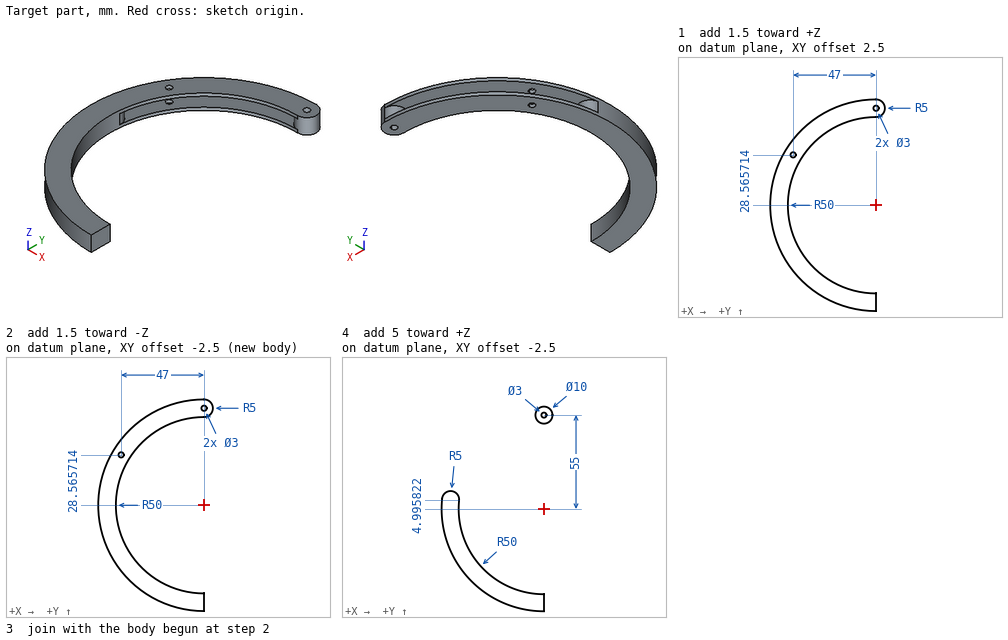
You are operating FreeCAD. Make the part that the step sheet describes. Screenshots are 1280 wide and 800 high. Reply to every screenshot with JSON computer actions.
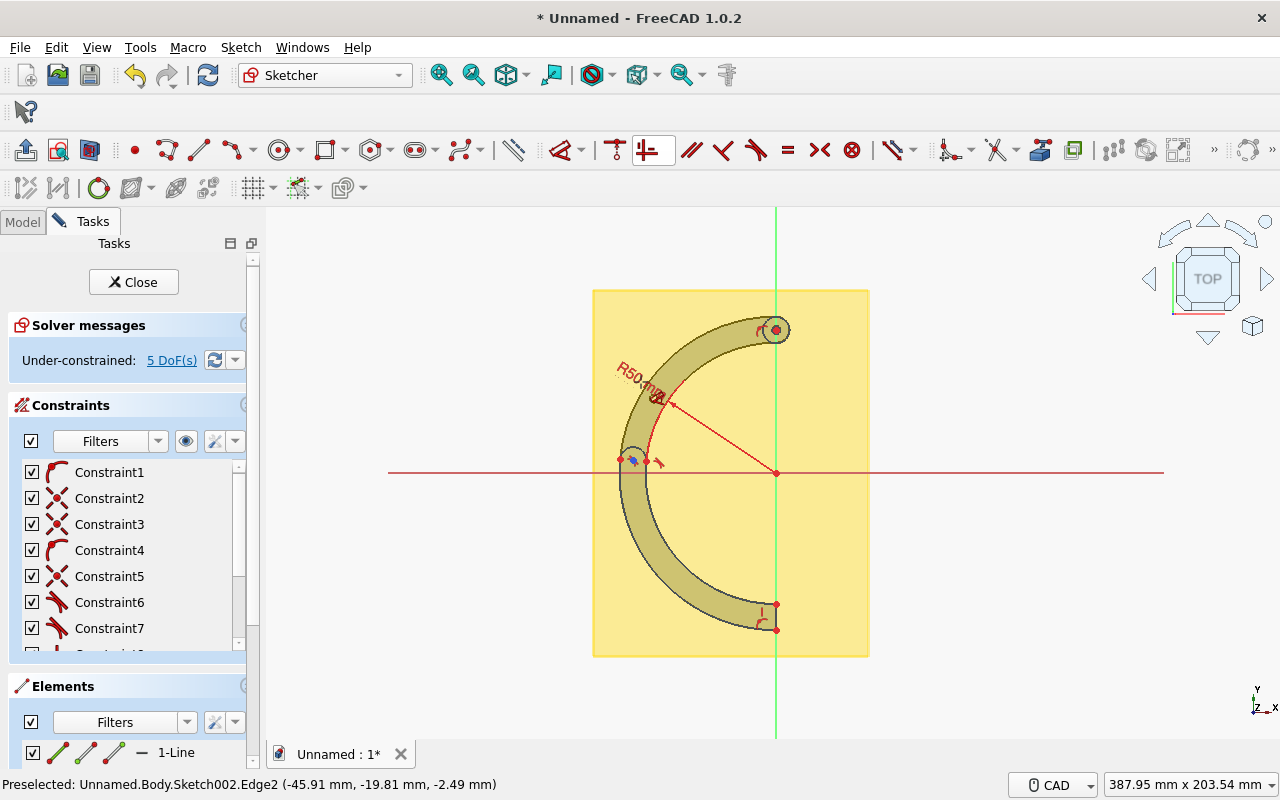
{"action": "scroll", "coordinate": [642, 450], "scroll_direction": "up", "scroll_amount": 6}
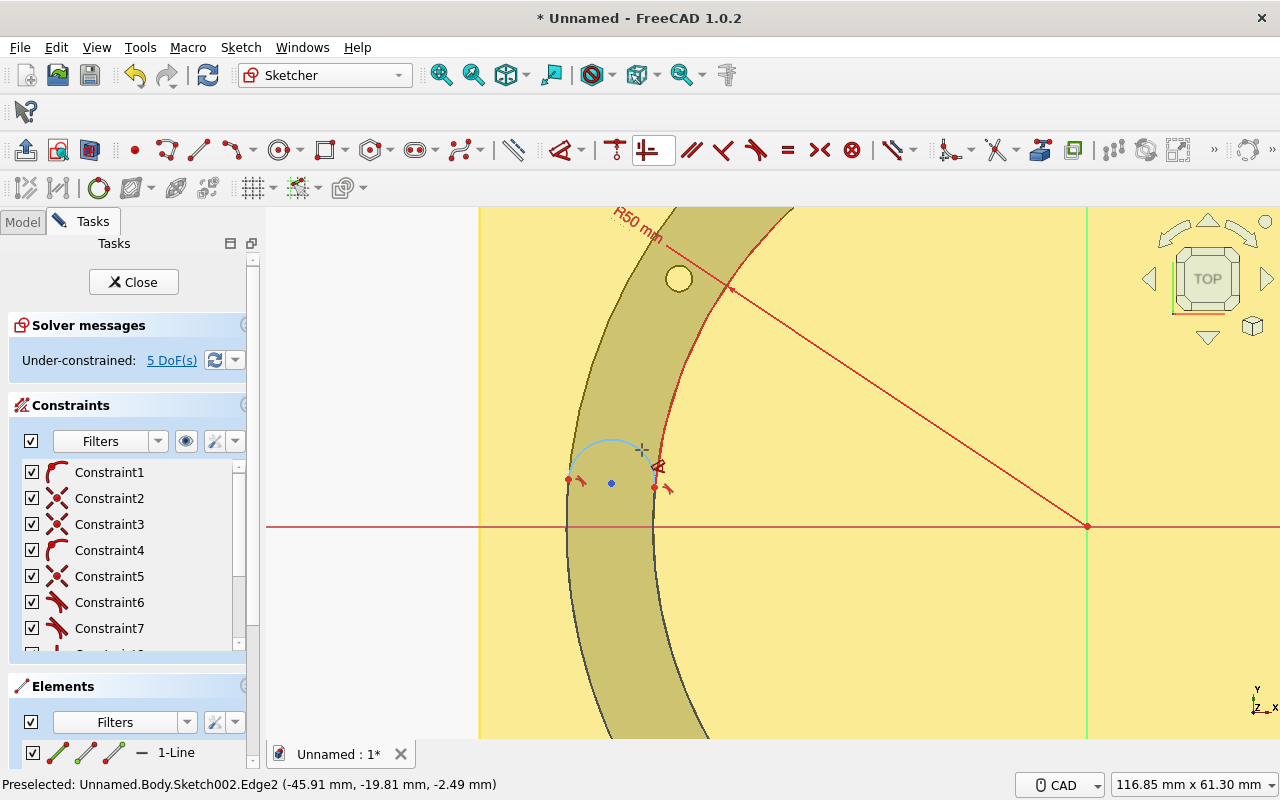
{"action": "left_click", "coordinate": [640, 450]}
{"action": "left_click", "coordinate": [661, 426]}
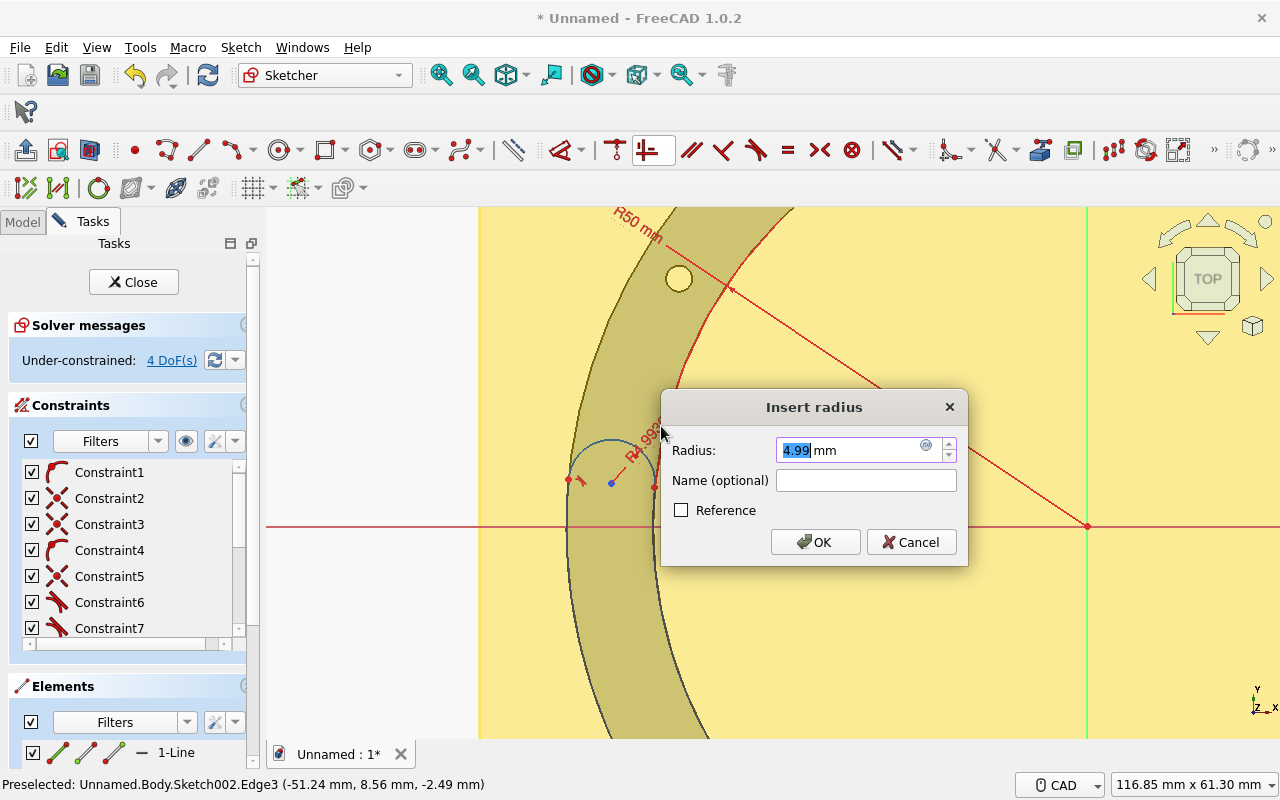
{"action": "type", "text": "5"}
{"action": "key", "text": "Return"}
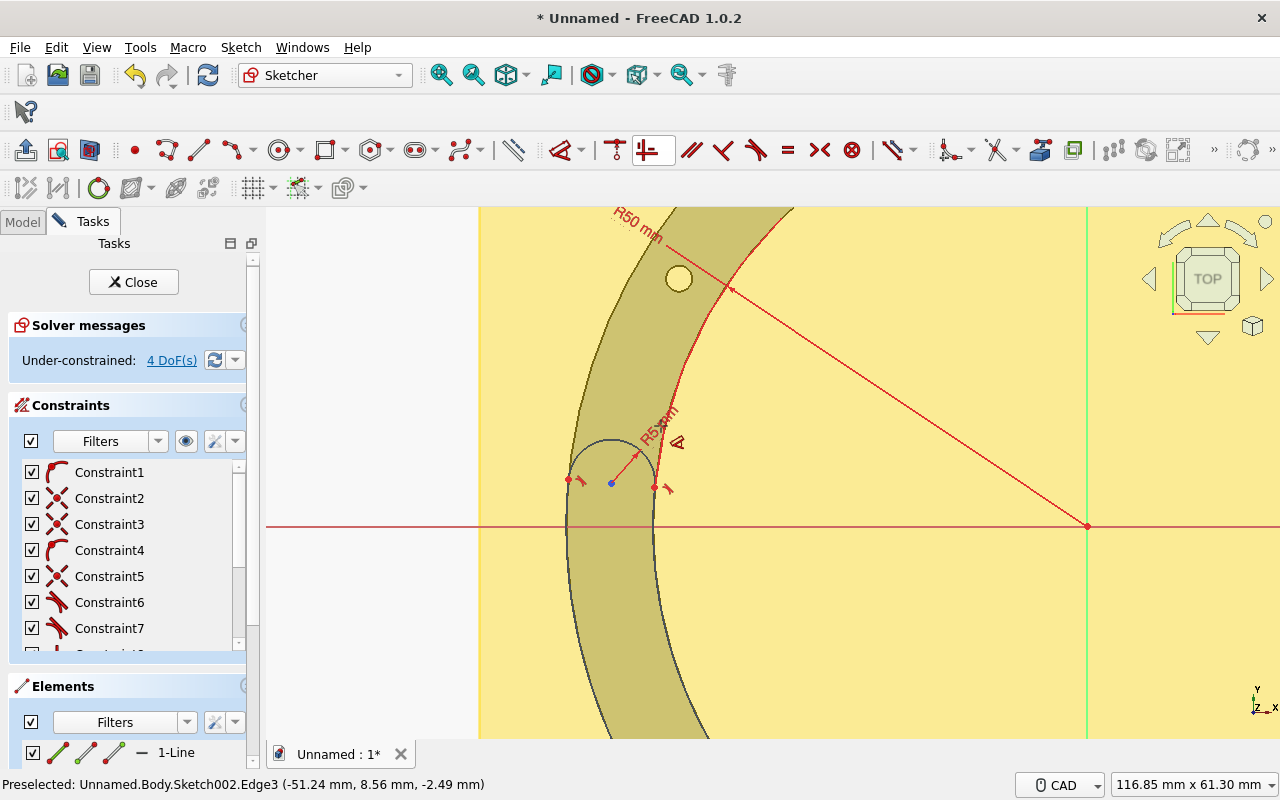
{"action": "scroll", "coordinate": [642, 450], "scroll_direction": "down", "scroll_amount": 6}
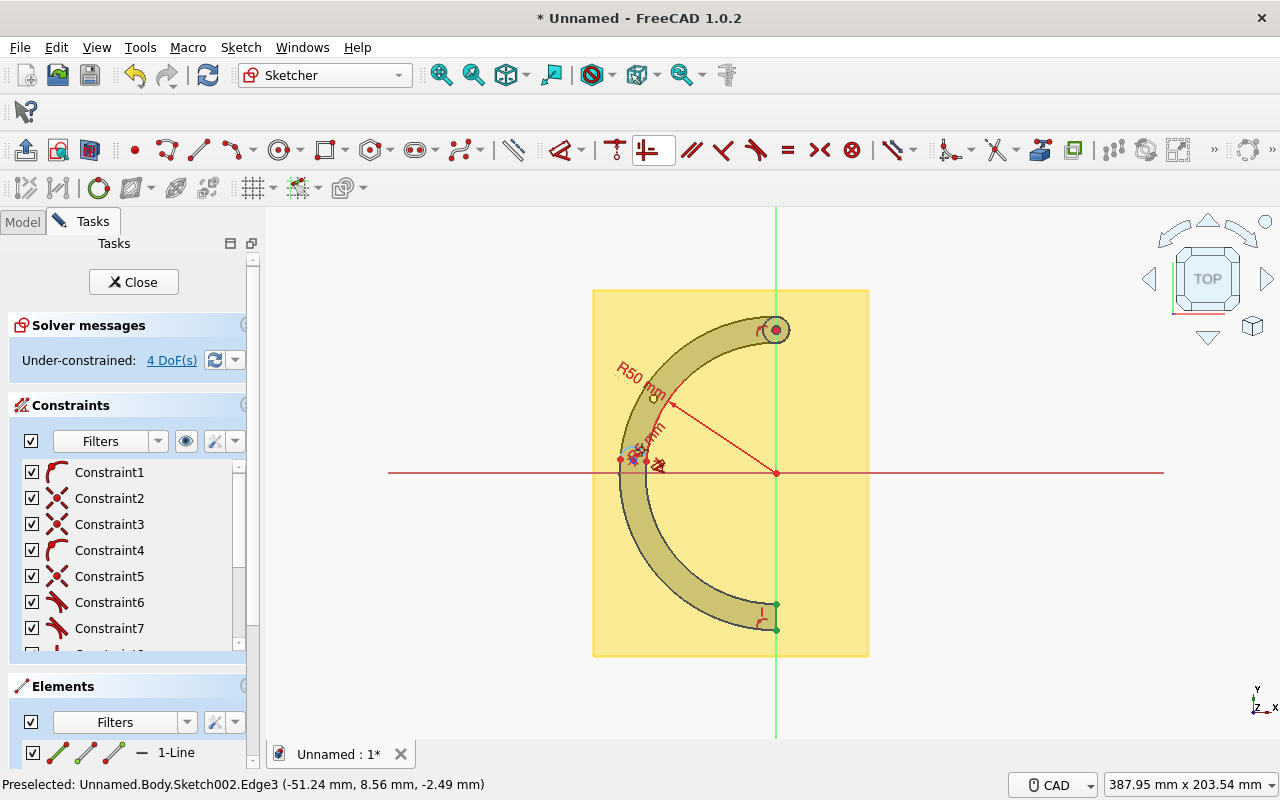
{"action": "scroll", "coordinate": [786, 321], "scroll_direction": "up", "scroll_amount": 3}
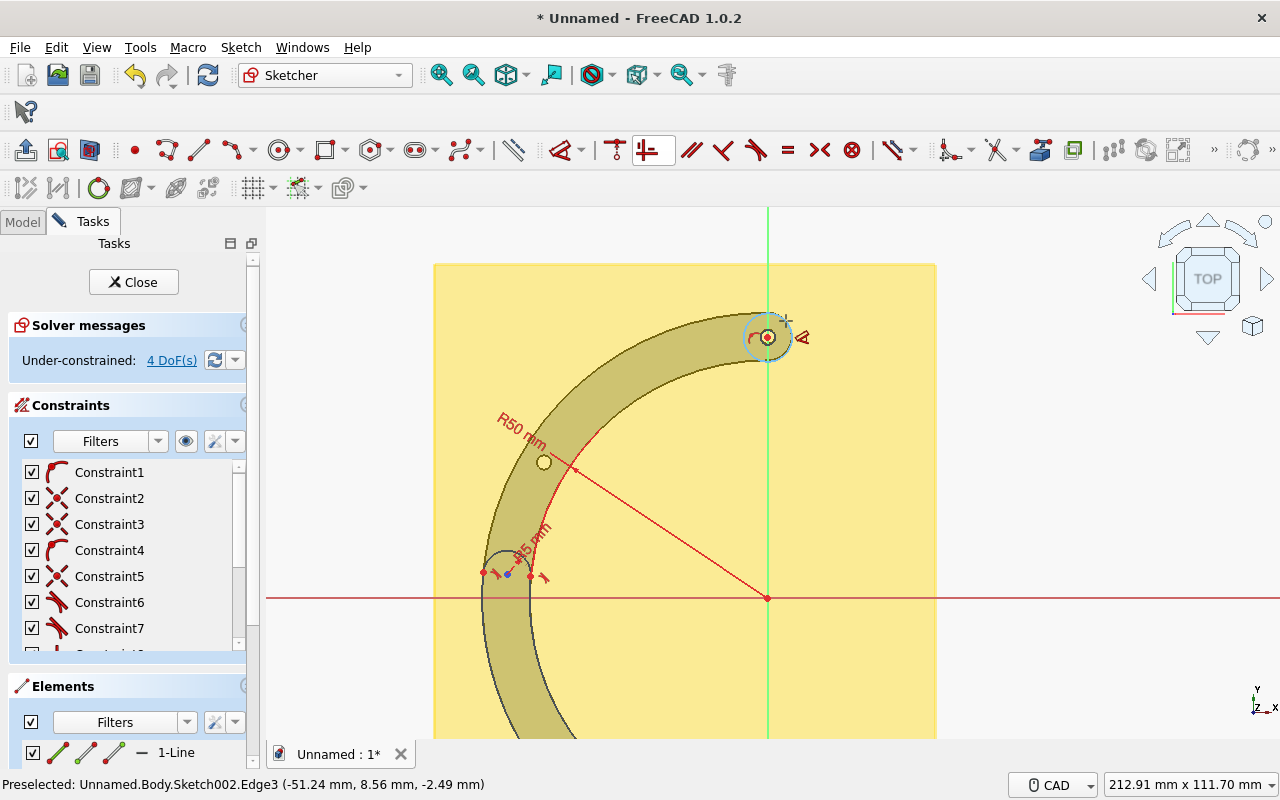
{"action": "left_click", "coordinate": [785, 320]}
{"action": "left_click", "coordinate": [807, 297]}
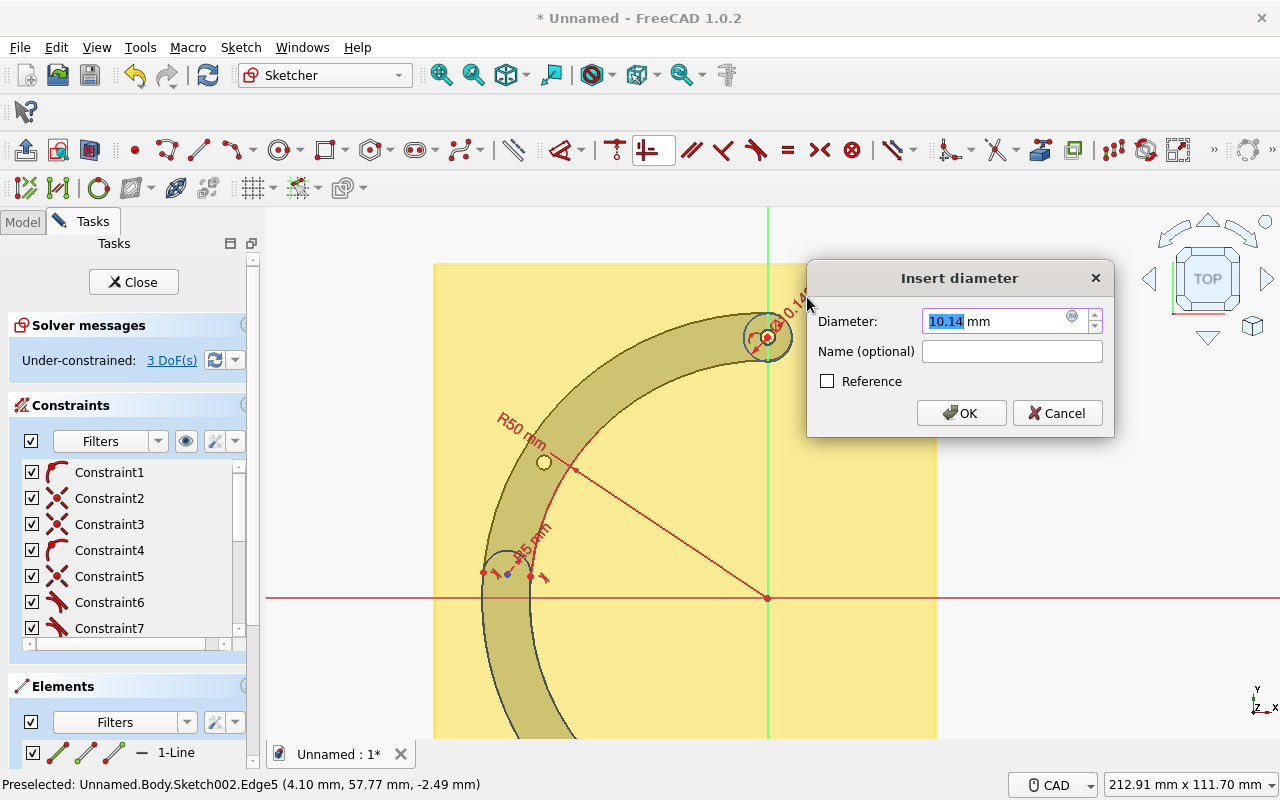
{"action": "type", "text": "10"}
{"action": "key", "text": "Return"}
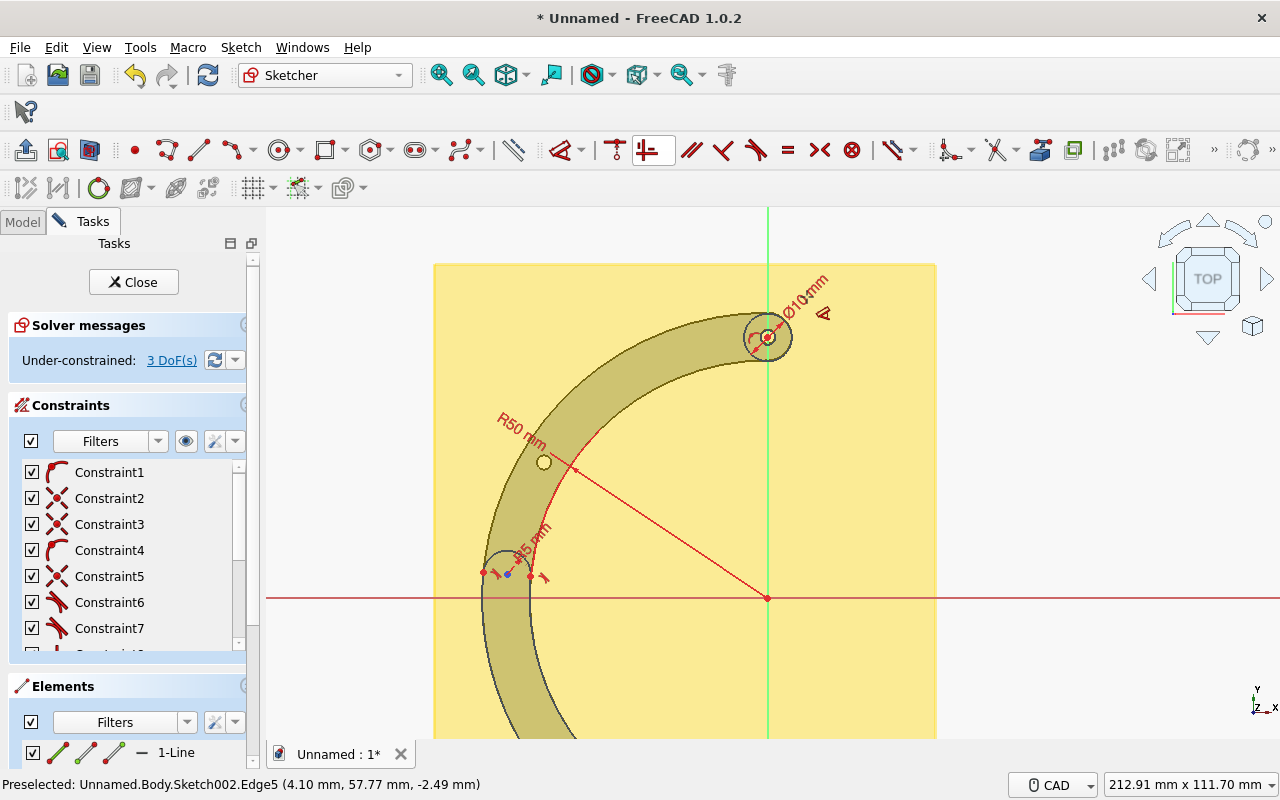
{"action": "scroll", "coordinate": [768, 330], "scroll_direction": "up", "scroll_amount": 6}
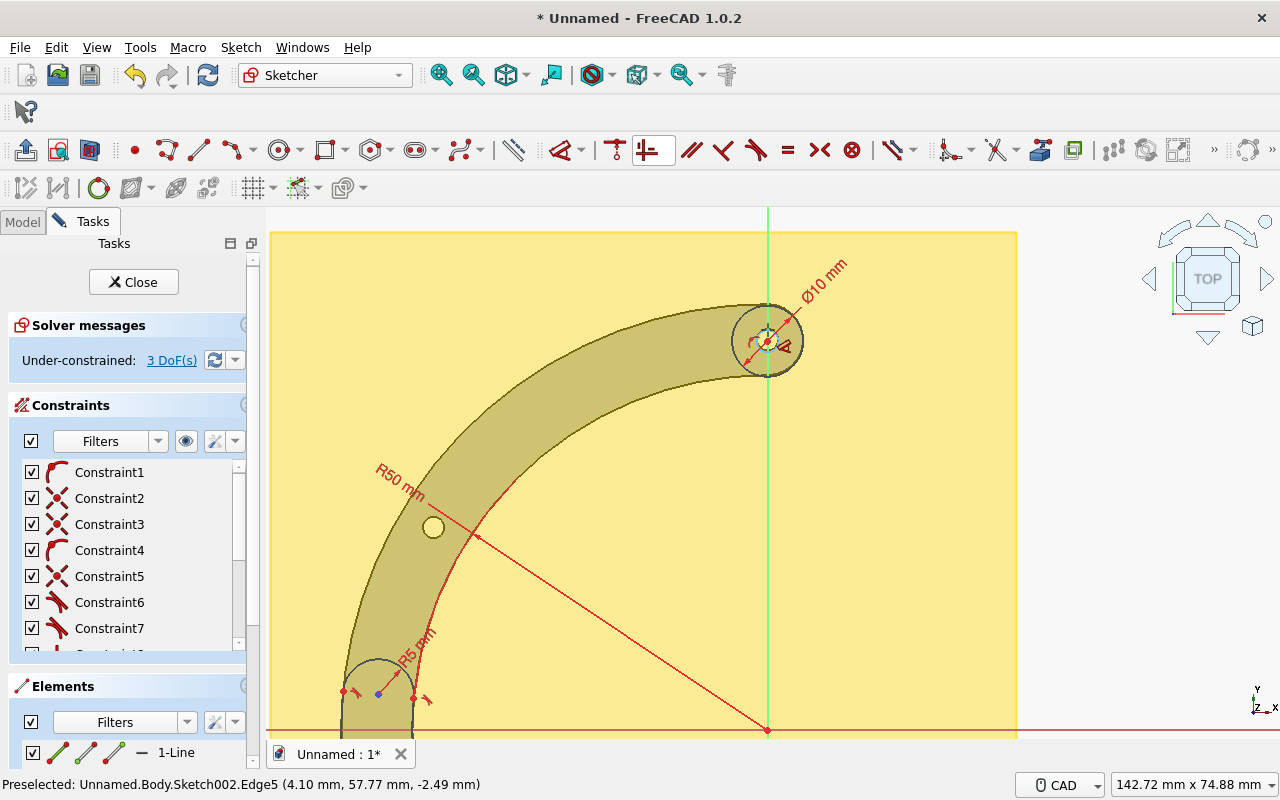
{"action": "left_click", "coordinate": [767, 330]}
{"action": "left_click", "coordinate": [795, 305]}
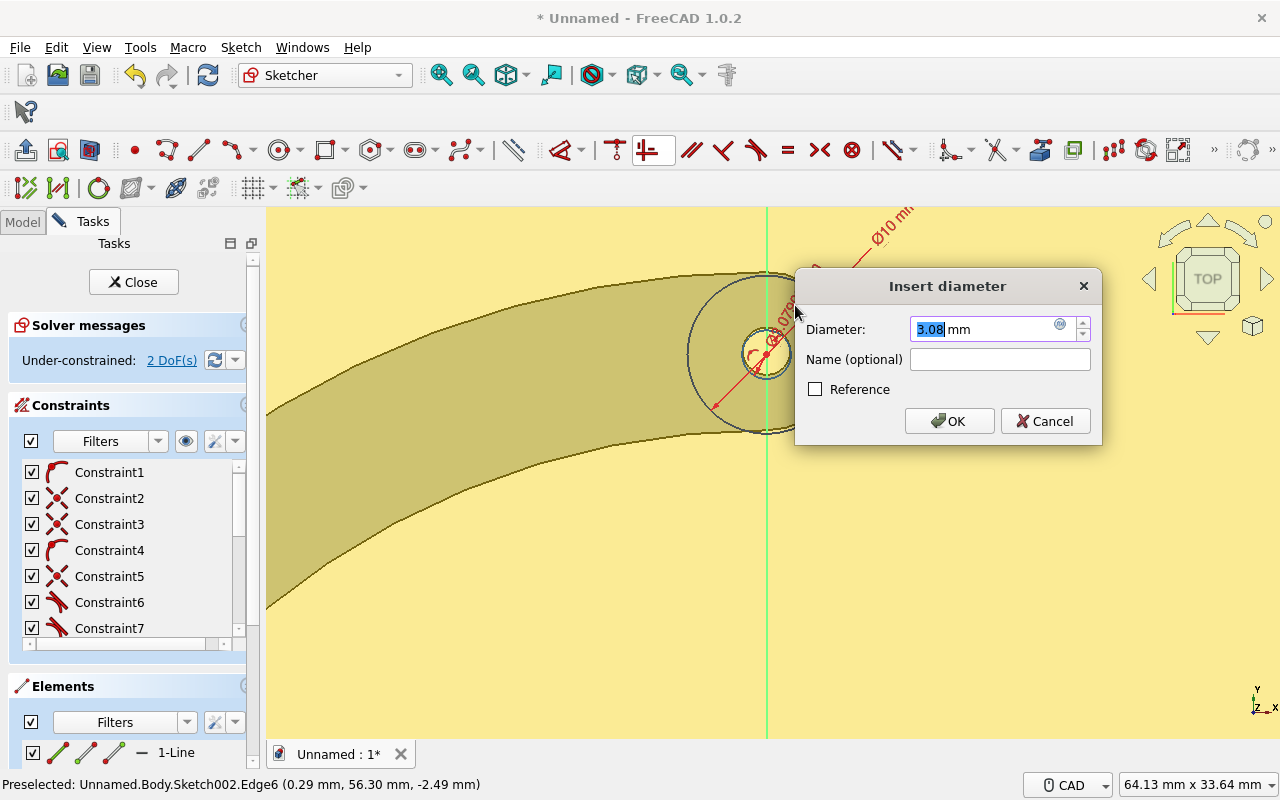
{"action": "type", "text": "3"}
{"action": "key", "text": "Return"}